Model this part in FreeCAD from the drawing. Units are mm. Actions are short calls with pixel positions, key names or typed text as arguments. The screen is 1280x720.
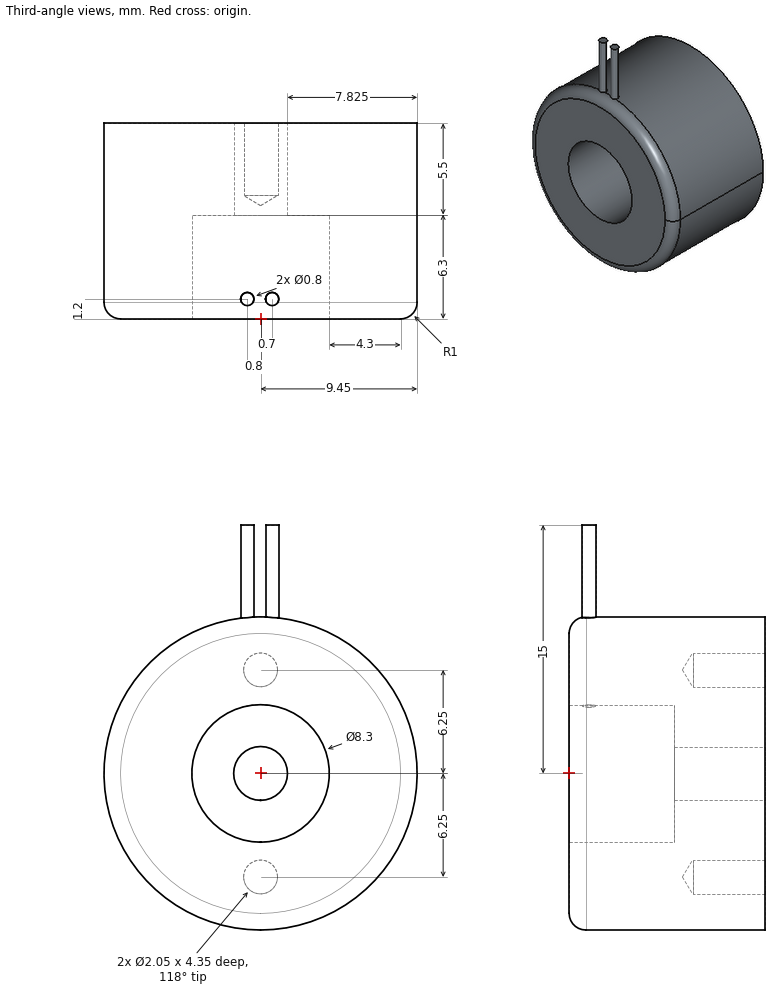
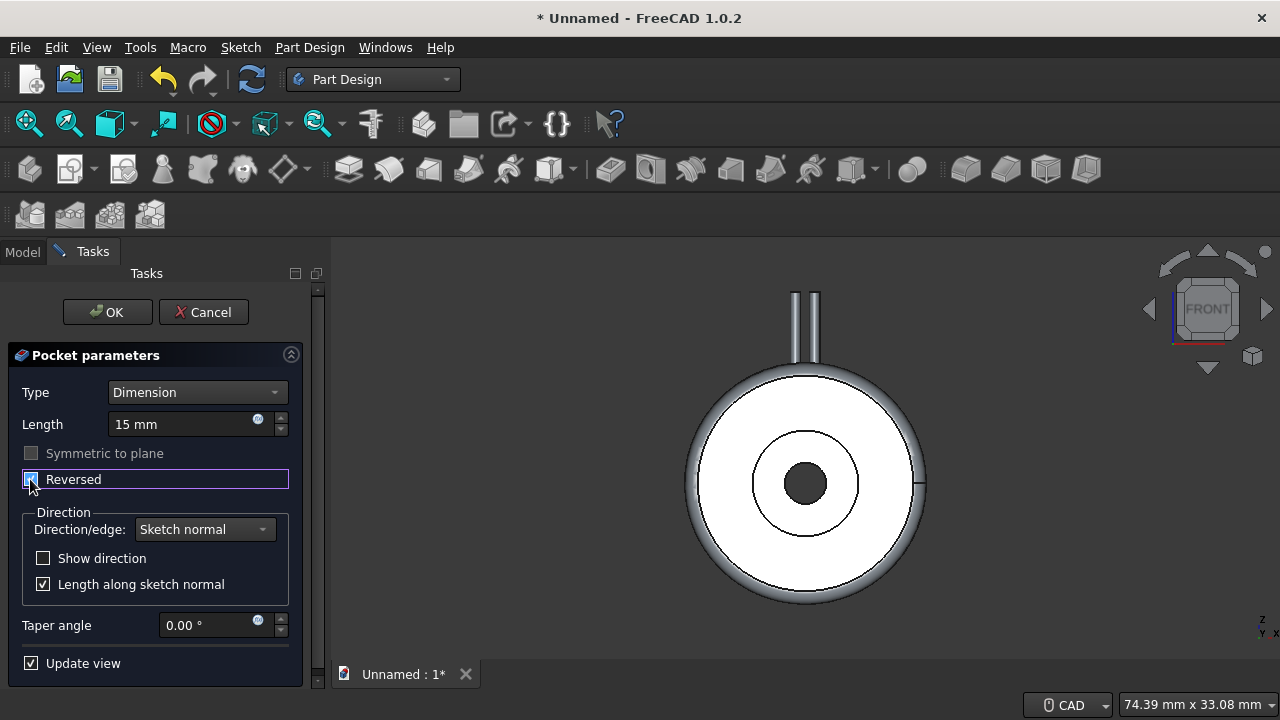
click(108, 312)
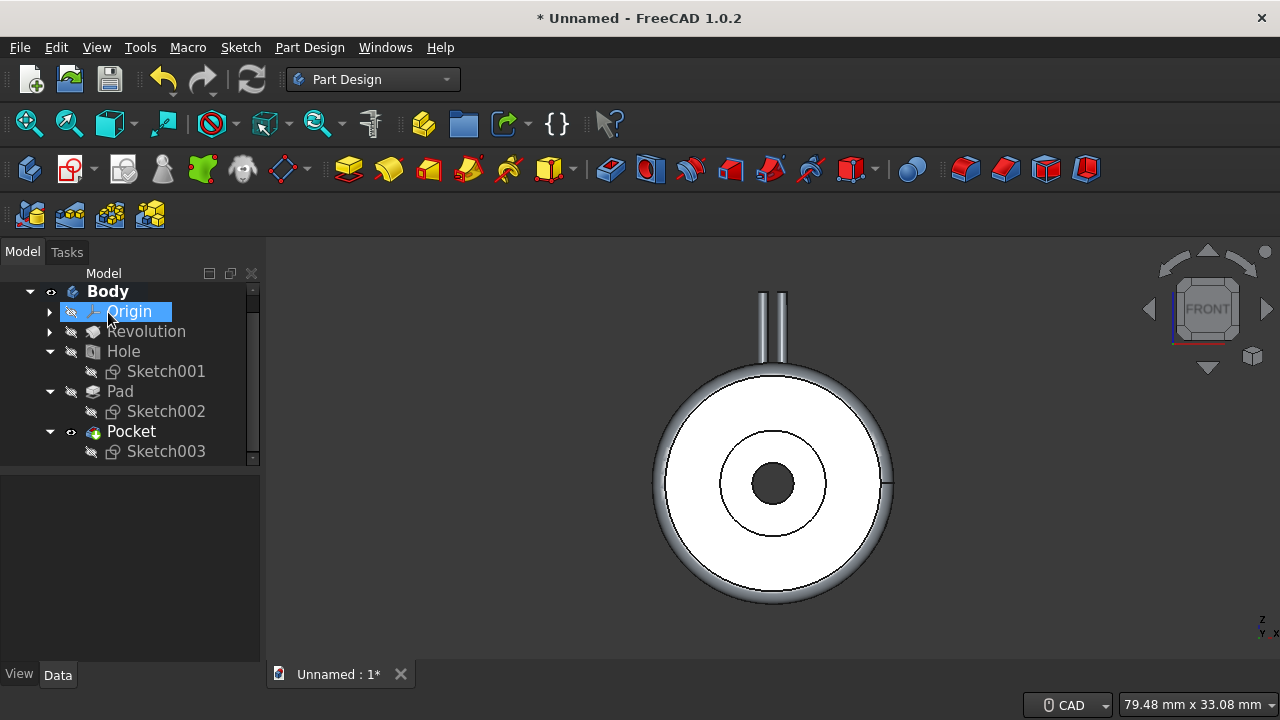
key(0)